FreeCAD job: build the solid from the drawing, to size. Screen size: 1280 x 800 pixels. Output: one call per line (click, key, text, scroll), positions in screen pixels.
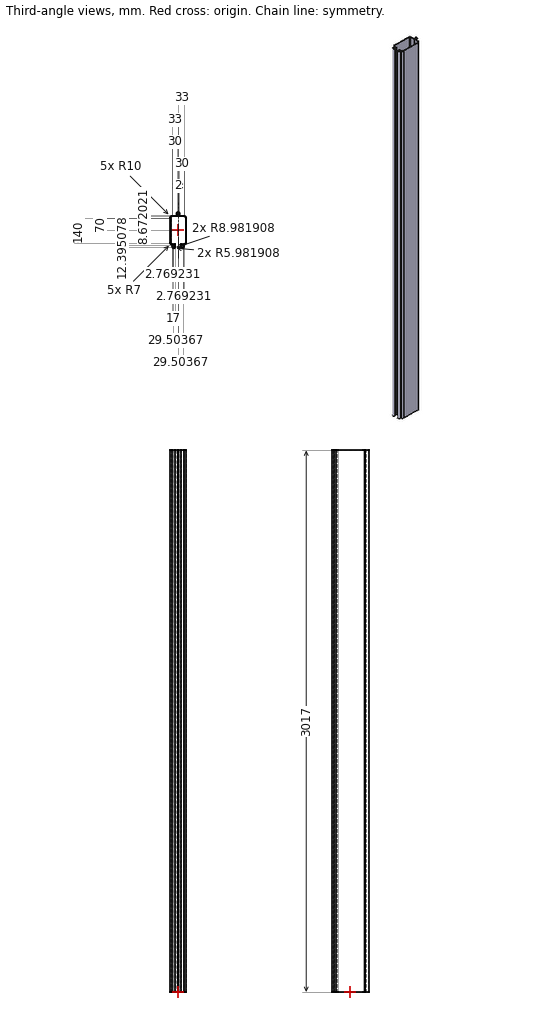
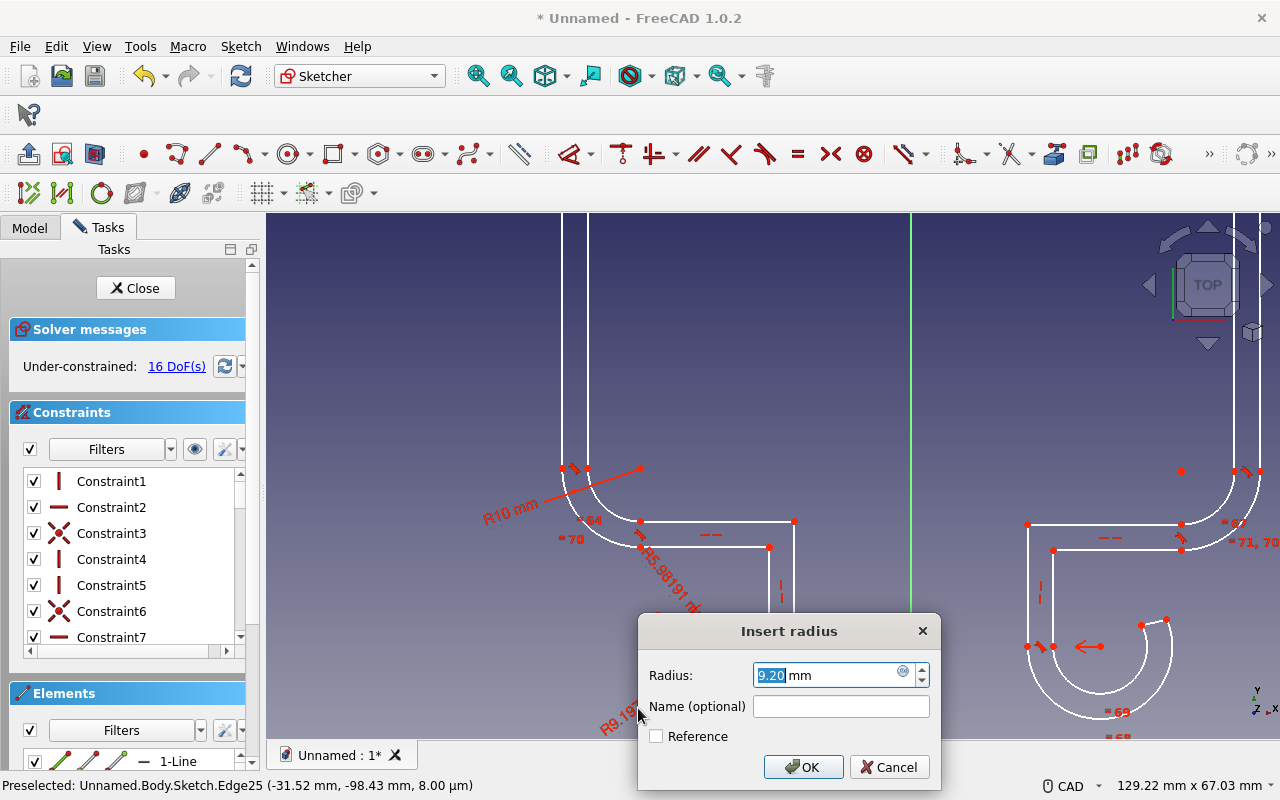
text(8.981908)
key(Return)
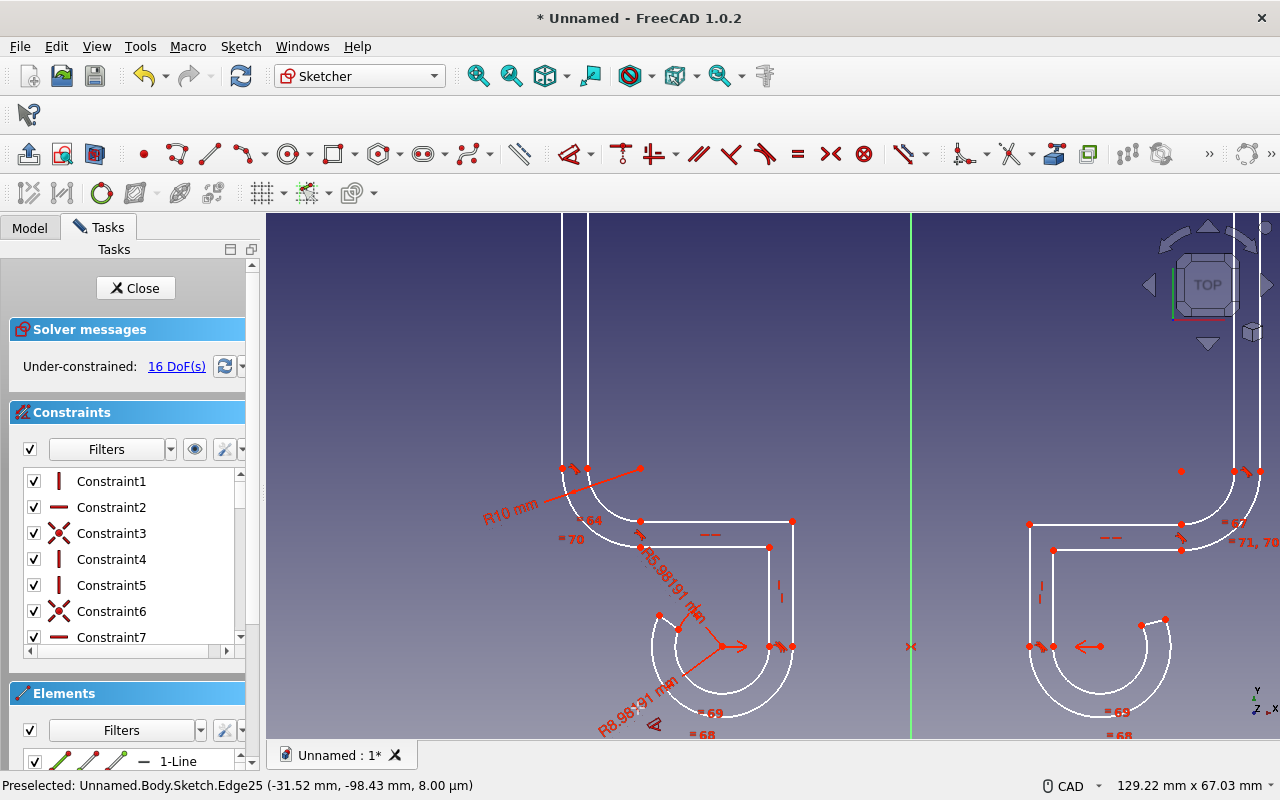
click(594, 493)
click(602, 394)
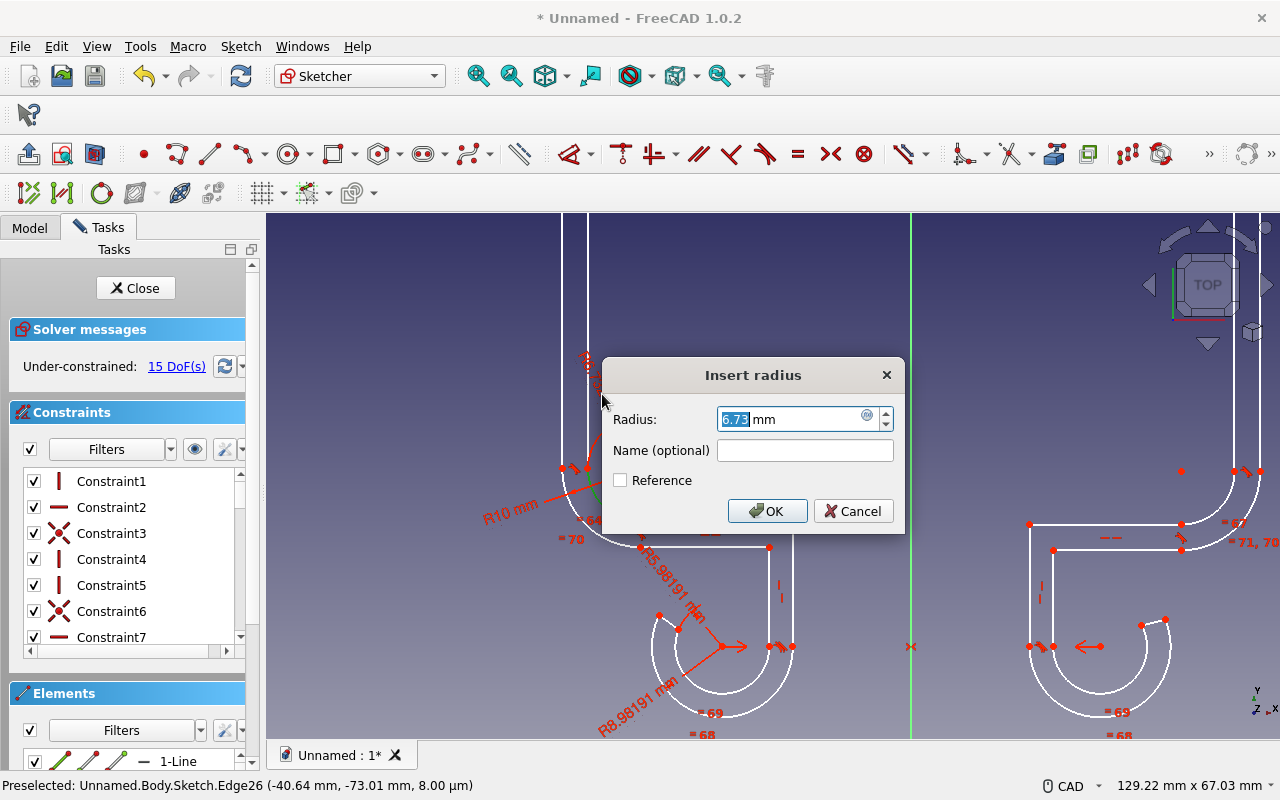
text(7)
key(Return)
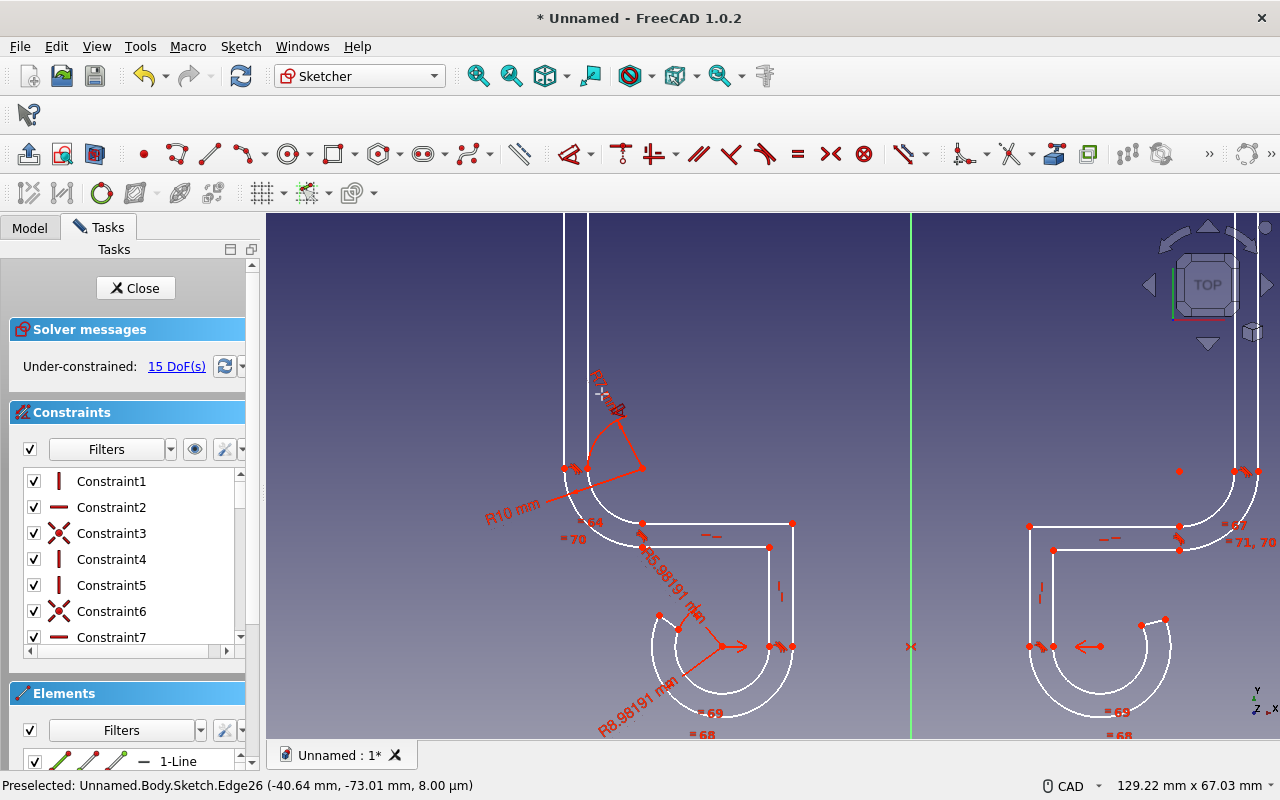
click(681, 547)
click(750, 581)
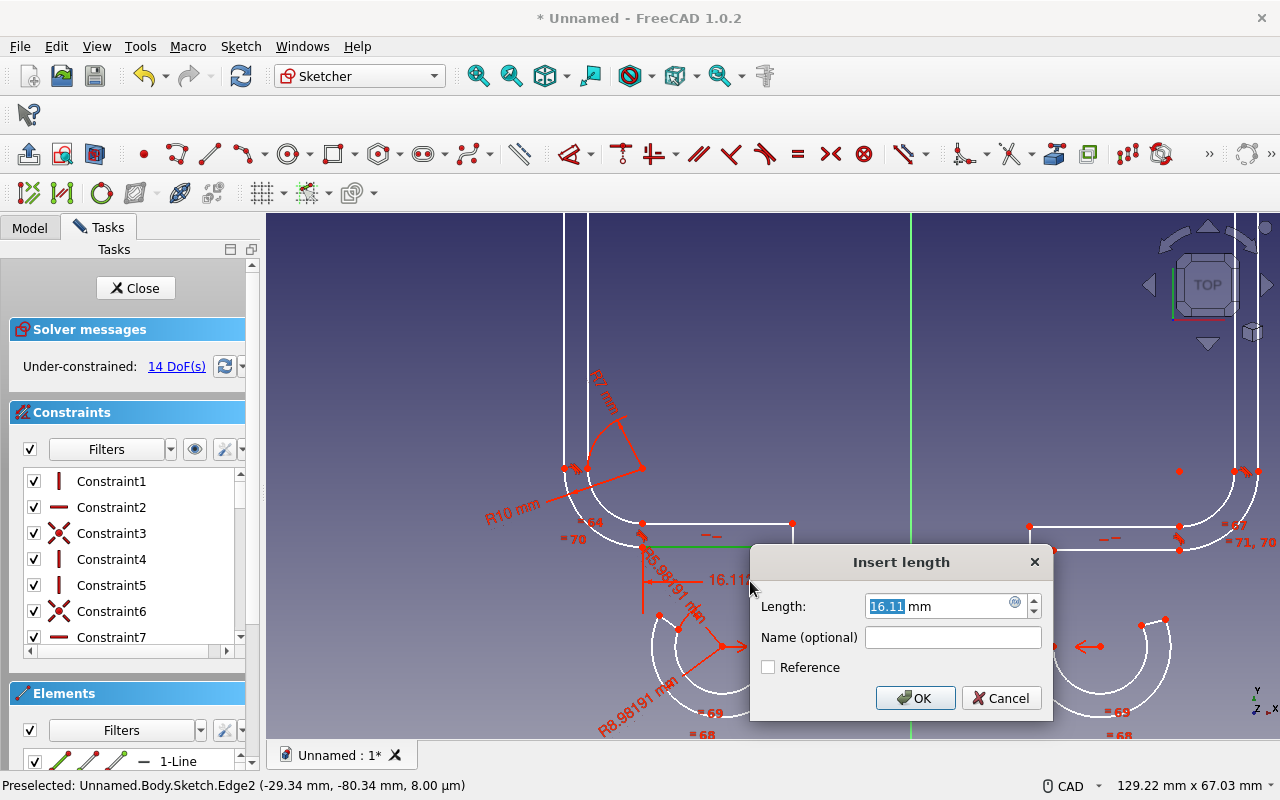
text(17)
key(Return)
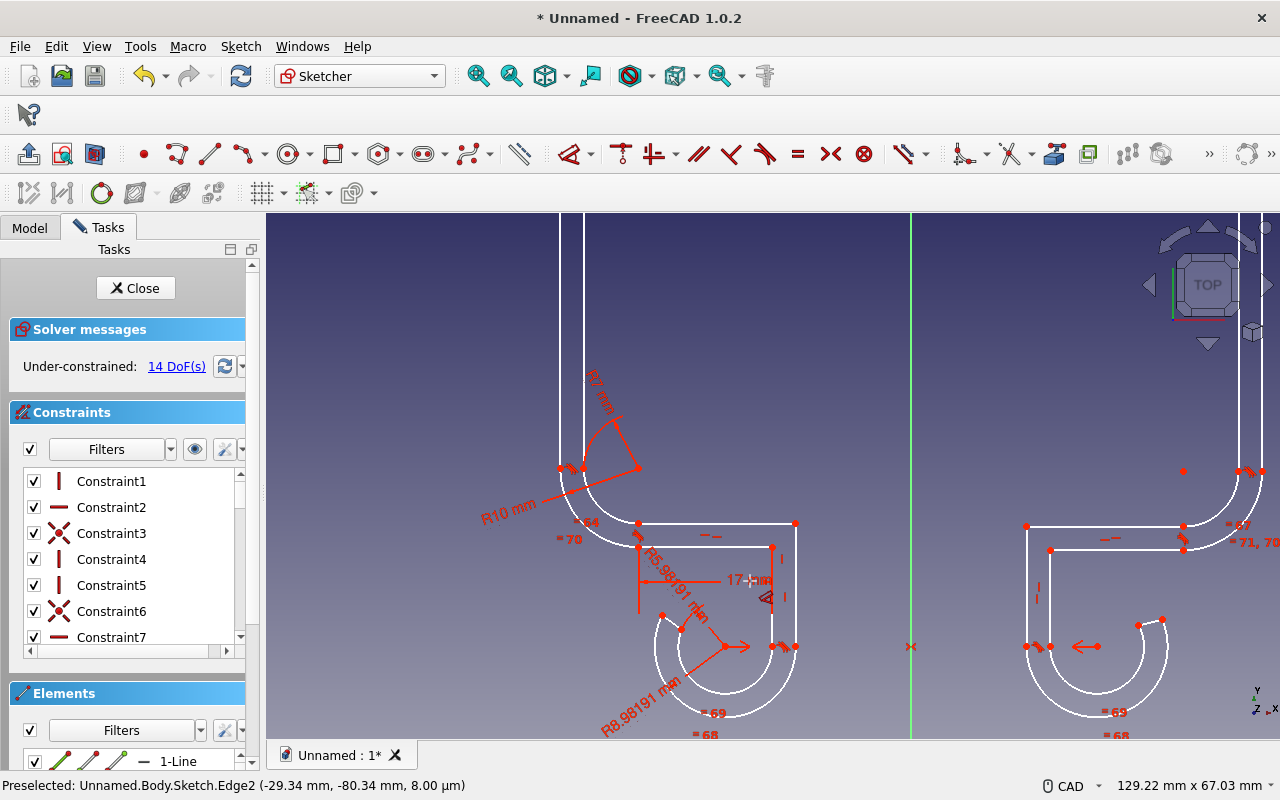
scroll(652, 619, down, 8)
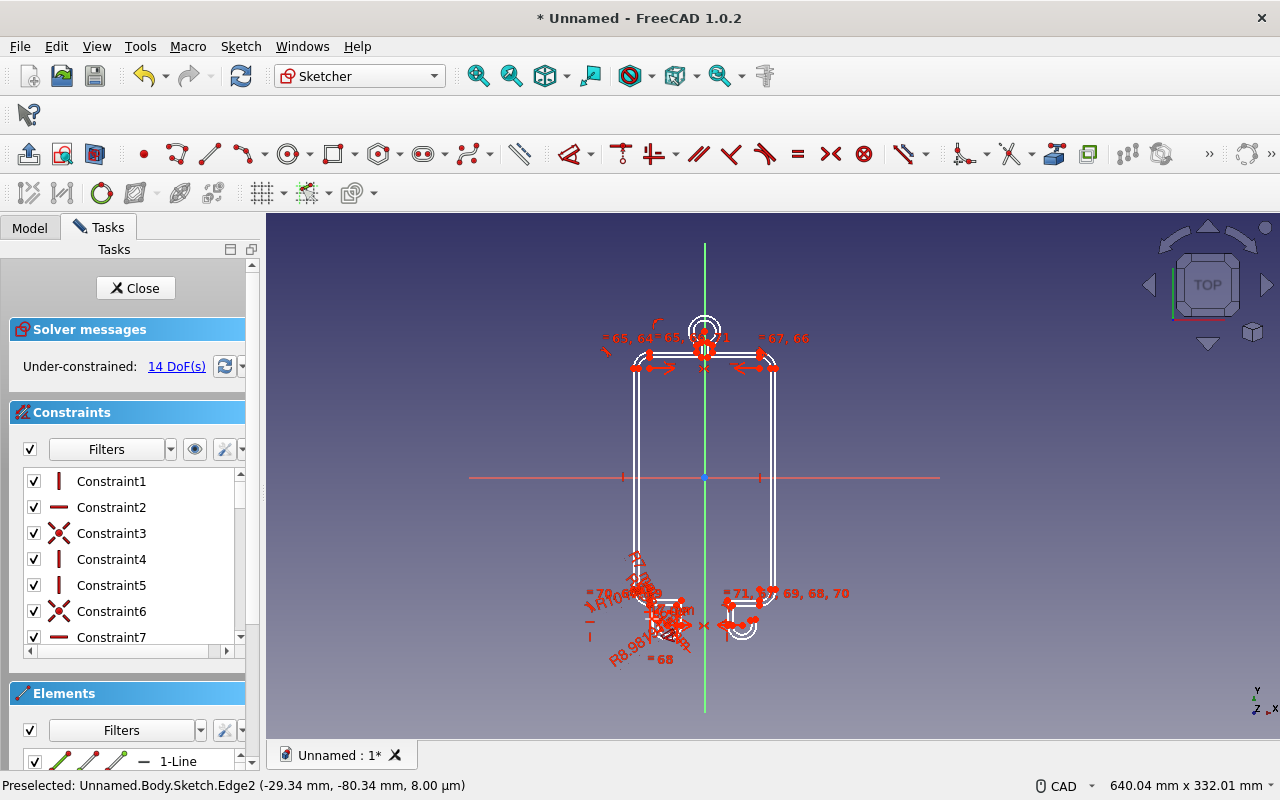
scroll(665, 357, up, 6)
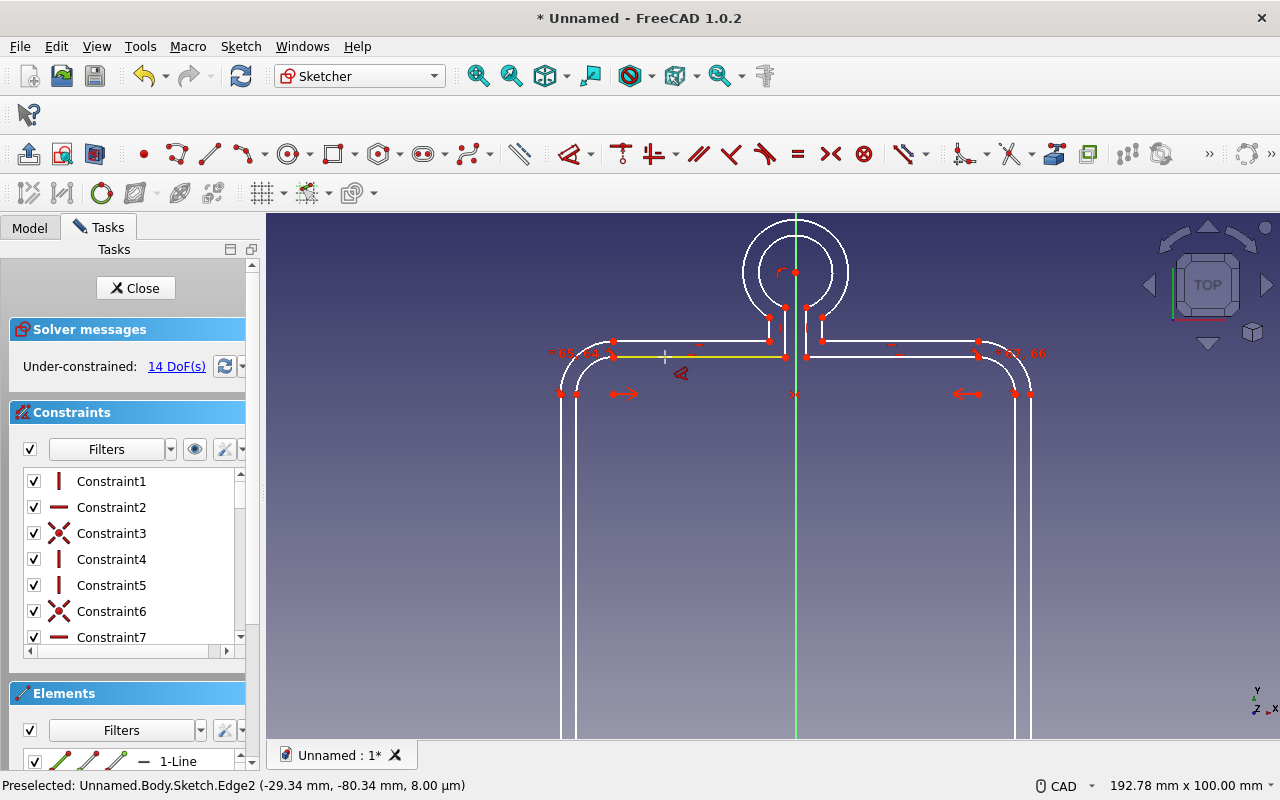
click(665, 357)
click(699, 323)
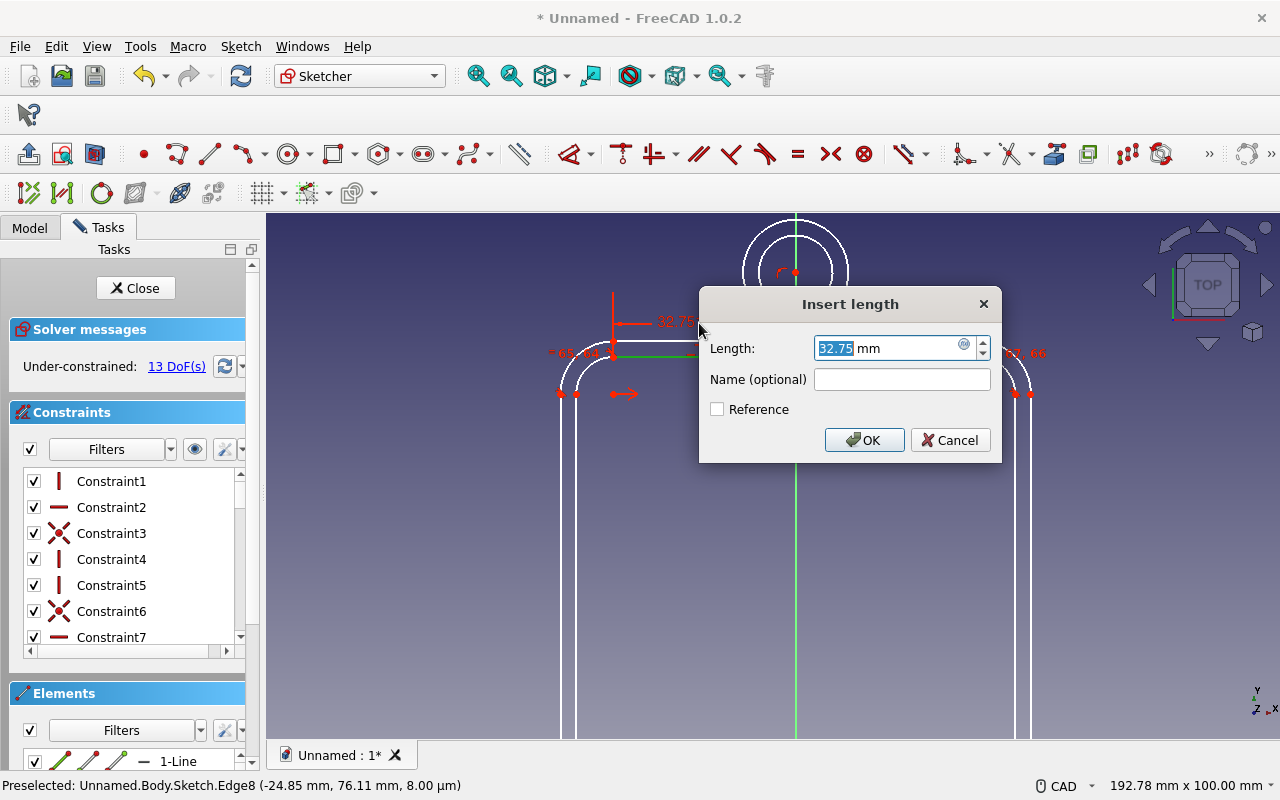
text(33)
key(Return)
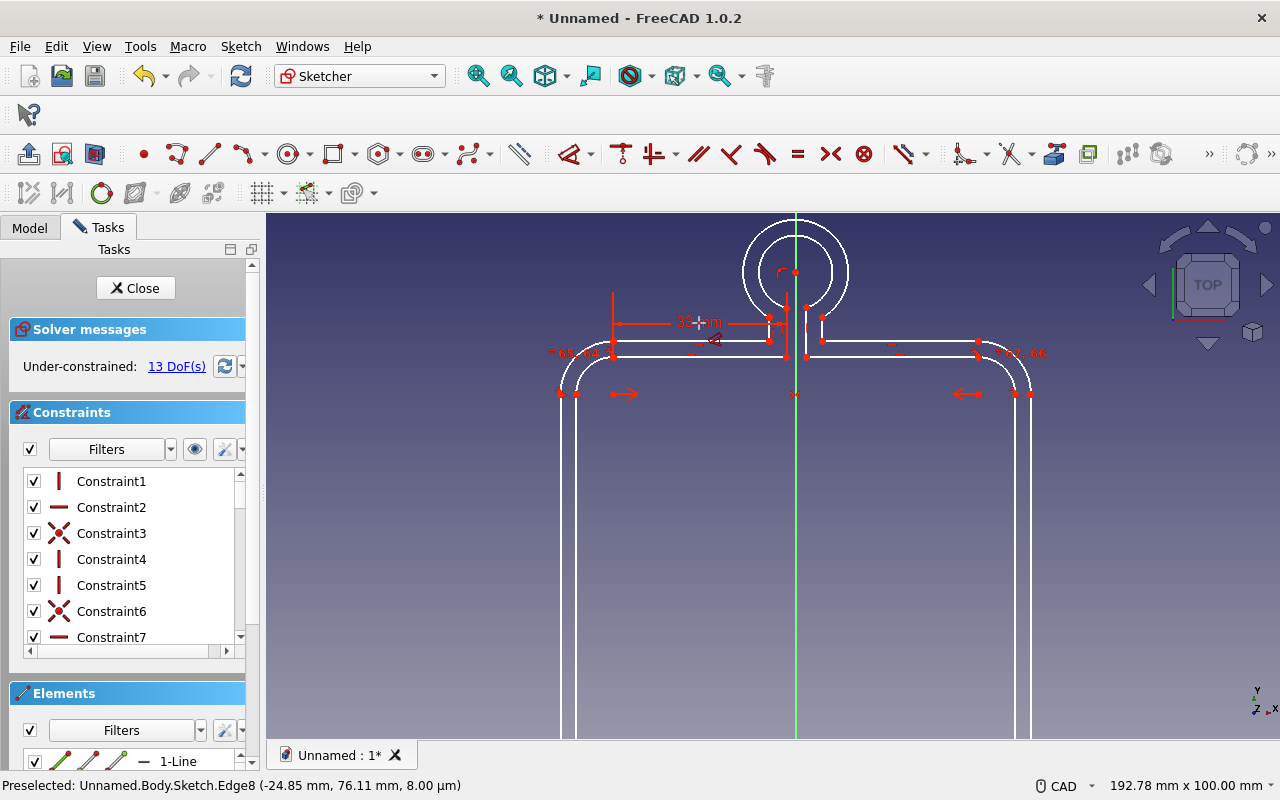
click(858, 357)
click(892, 323)